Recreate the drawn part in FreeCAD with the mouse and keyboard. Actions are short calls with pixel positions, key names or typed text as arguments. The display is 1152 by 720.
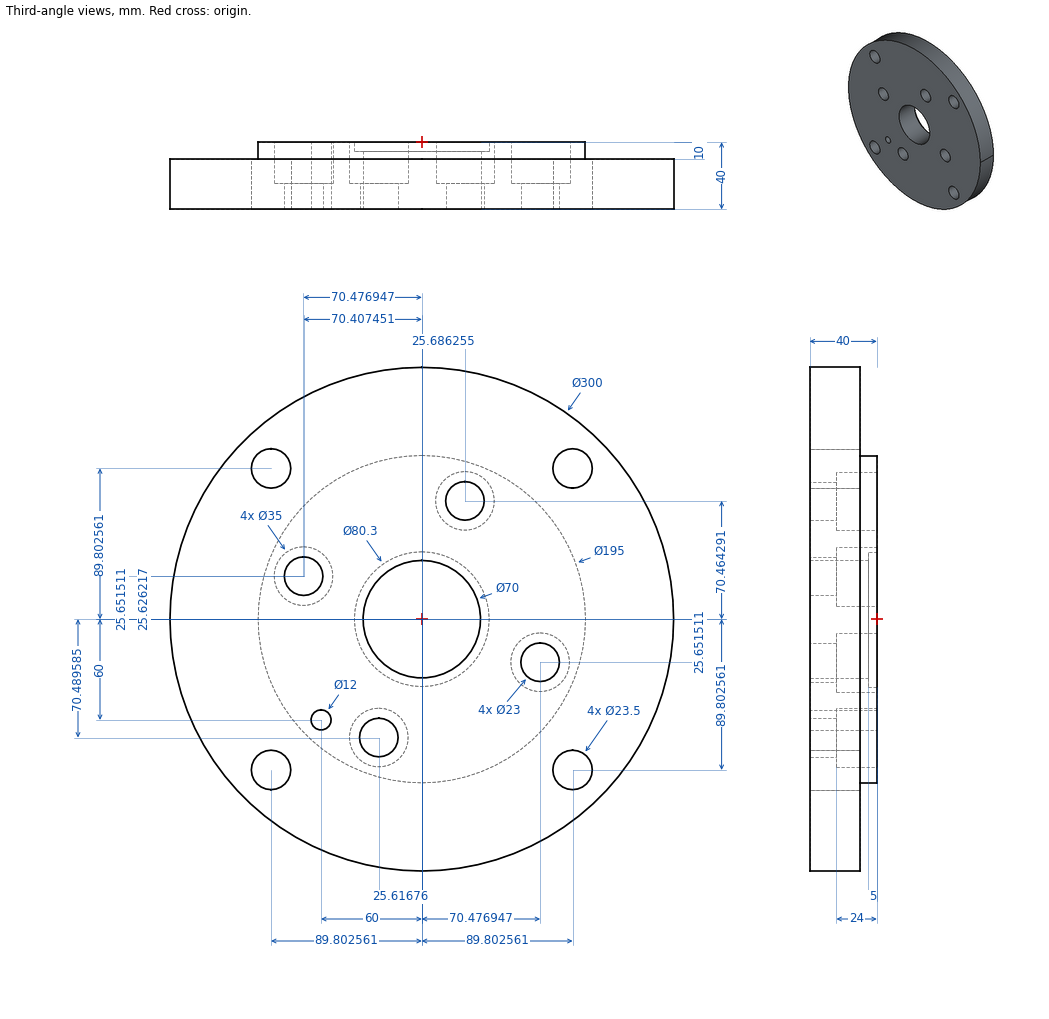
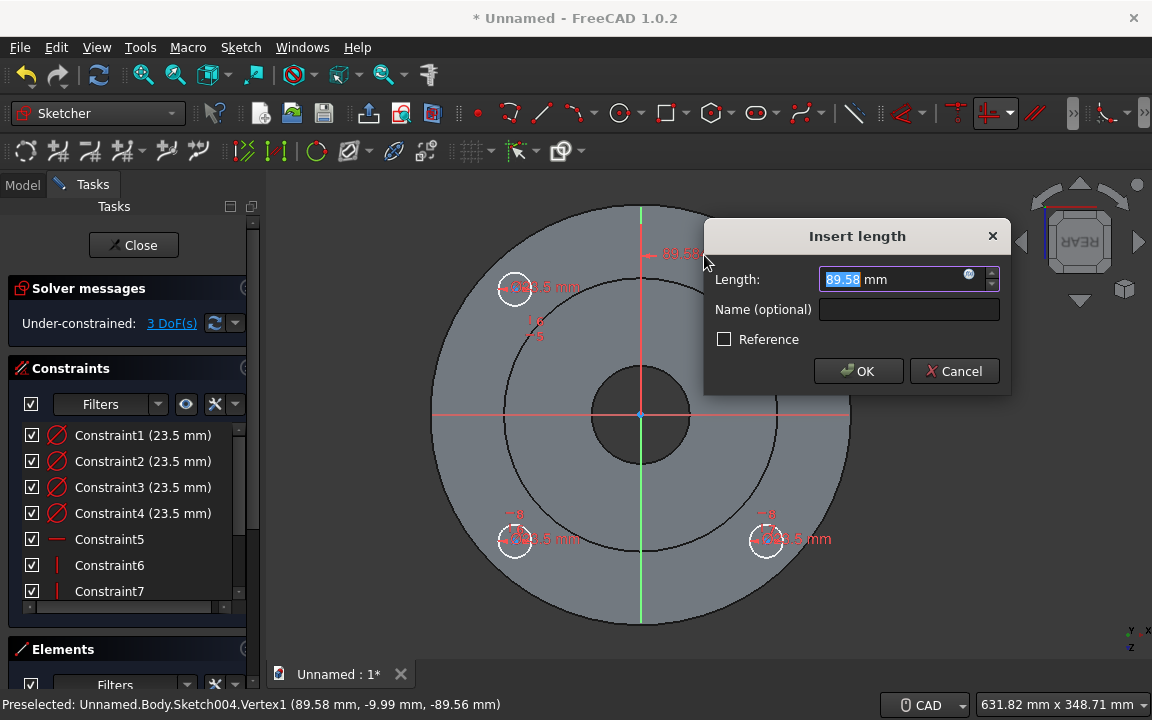
text(89.802561)
key(Return)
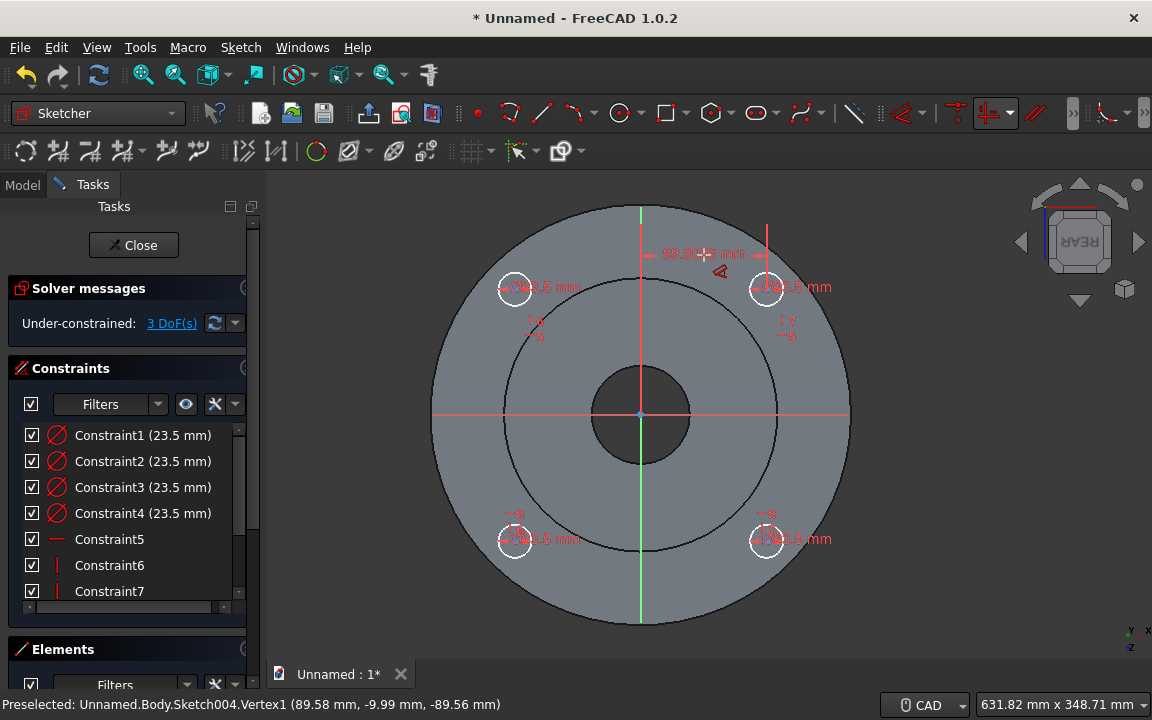
click(767, 289)
click(801, 352)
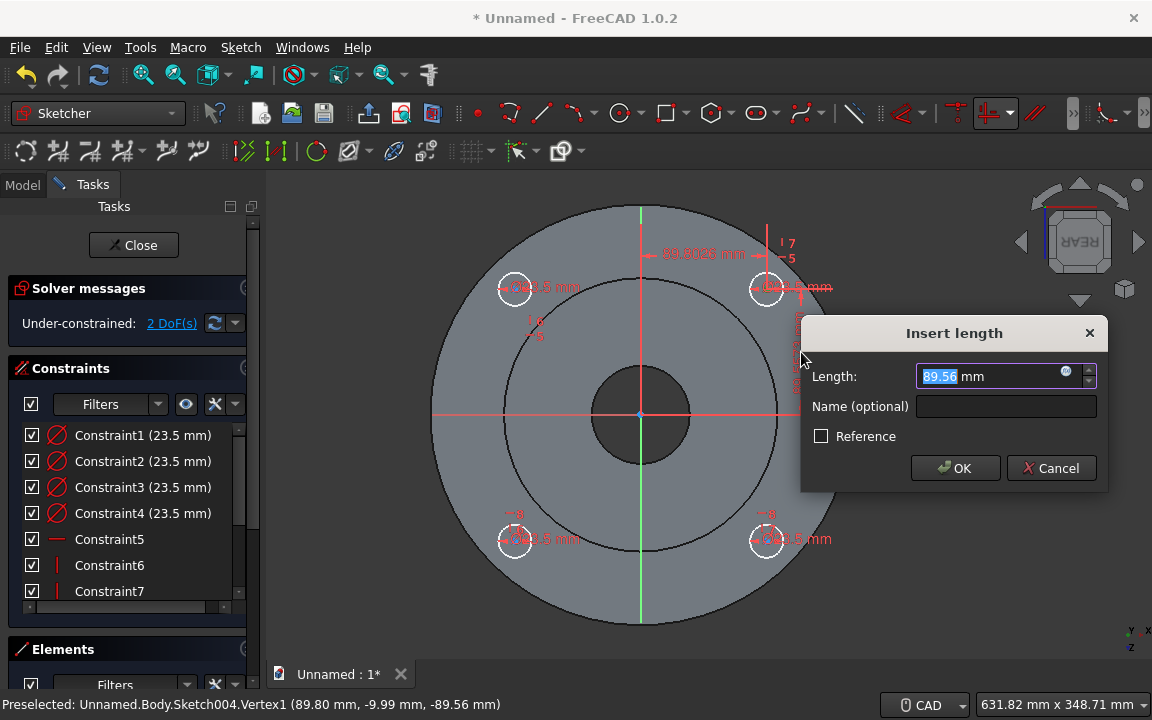
text(89.802561)
key(Return)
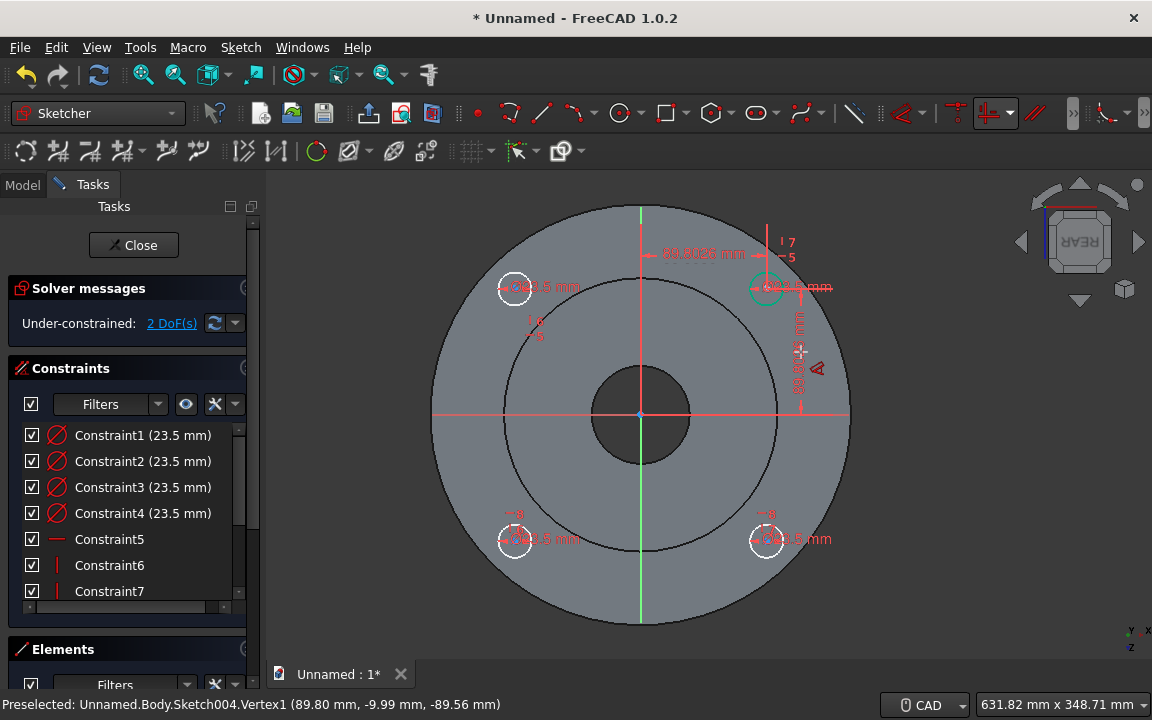
click(515, 289)
click(578, 255)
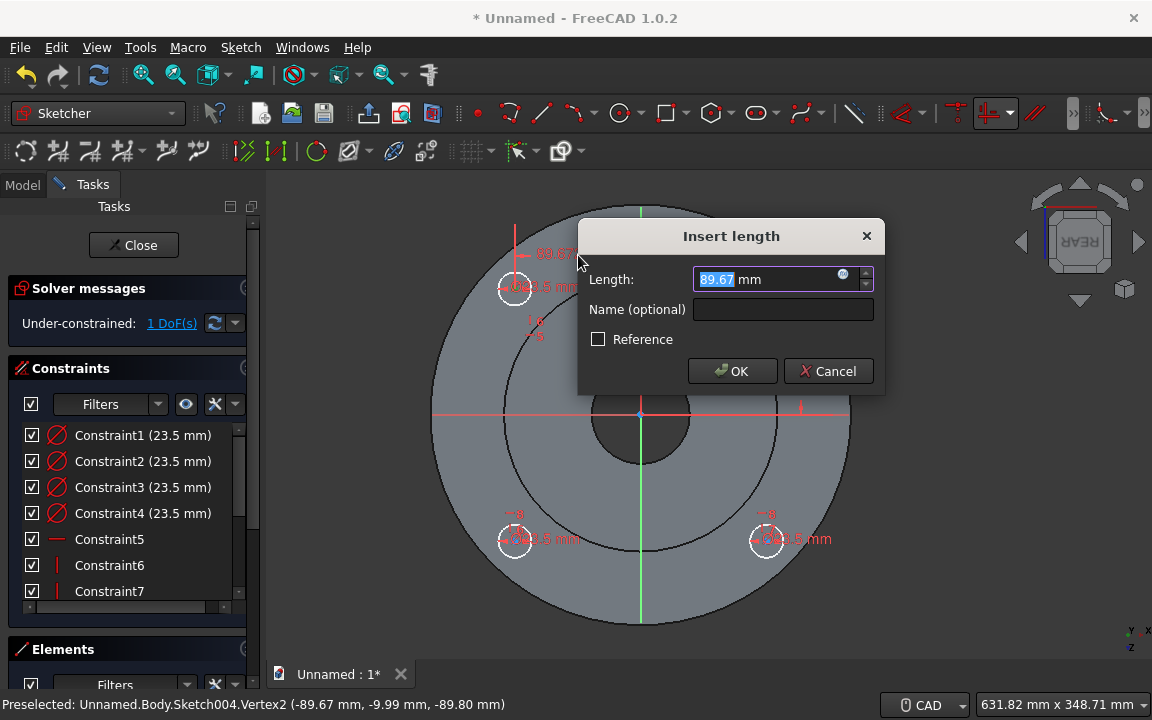
text(89.802561)
key(Return)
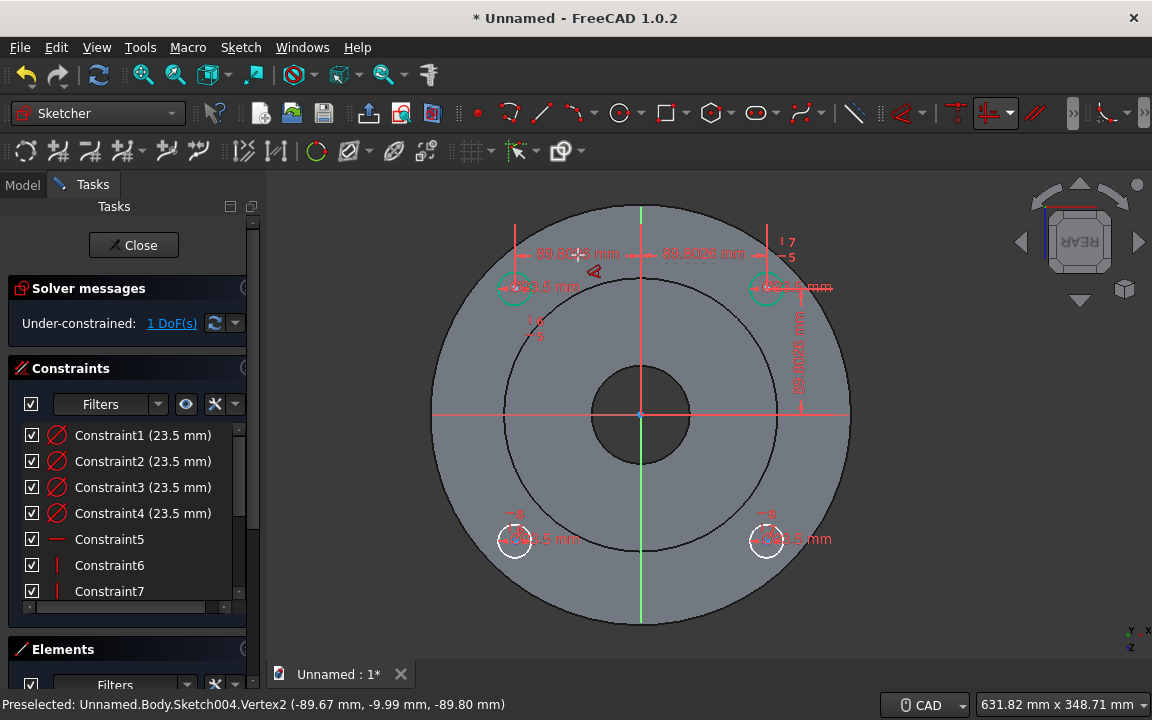
click(515, 541)
click(481, 478)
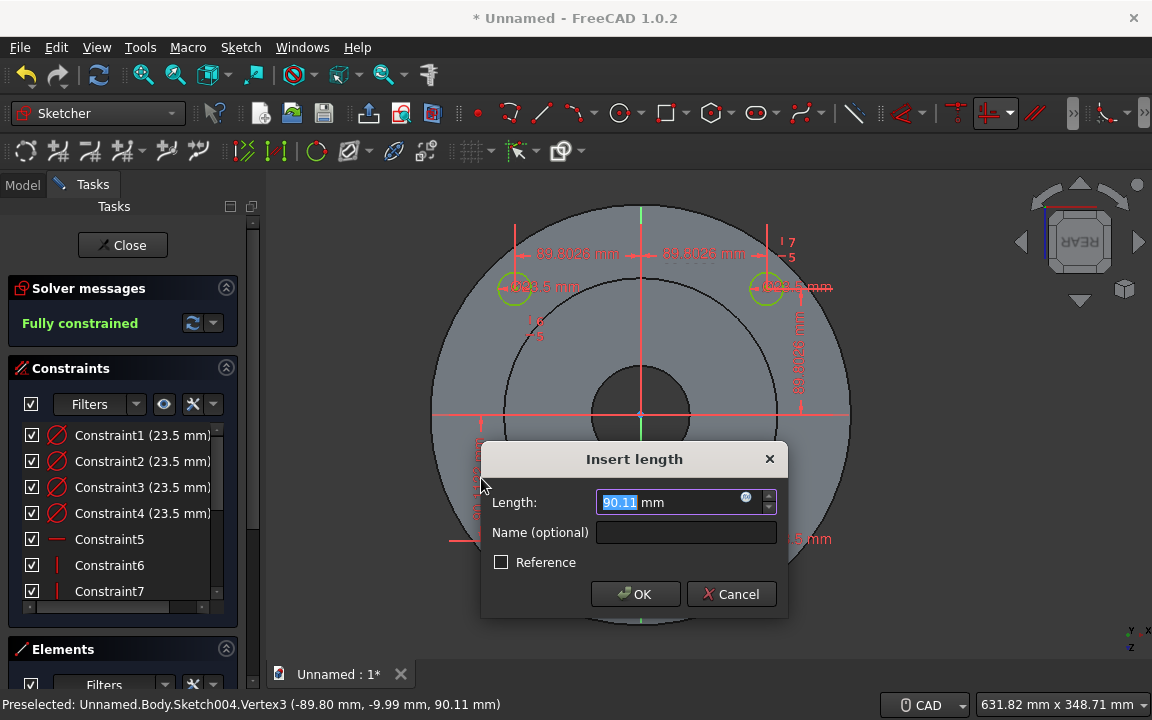
text(89.802561)
key(Return)
key(Escape)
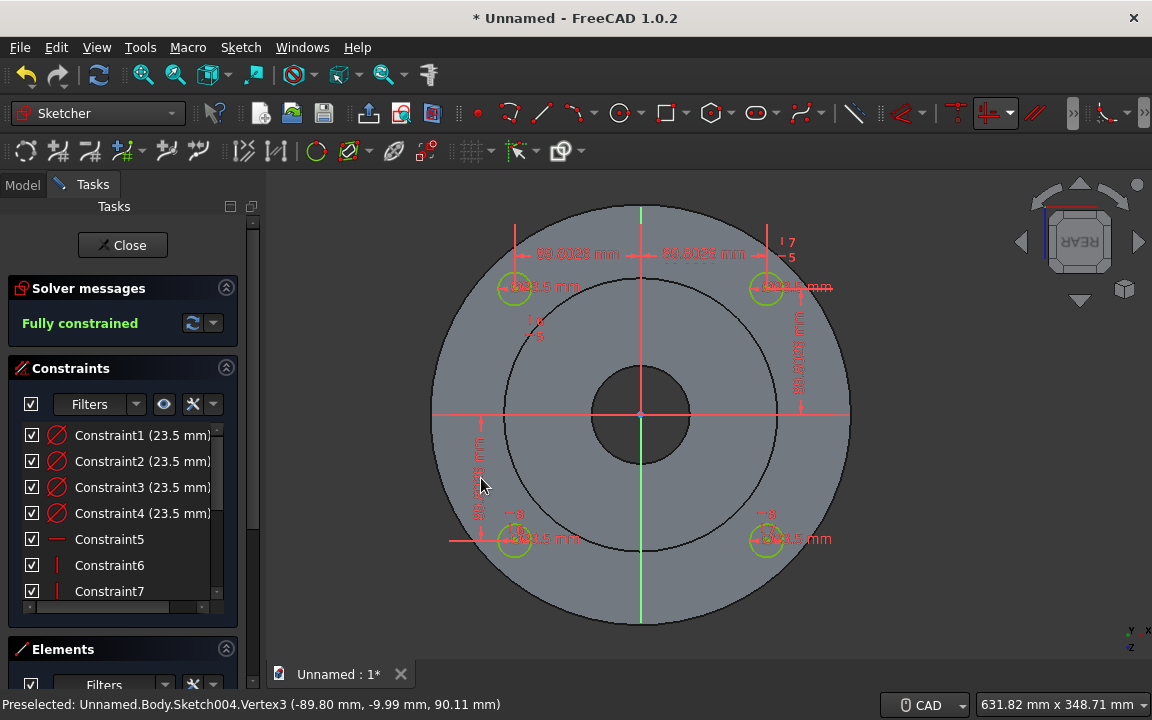
click(123, 245)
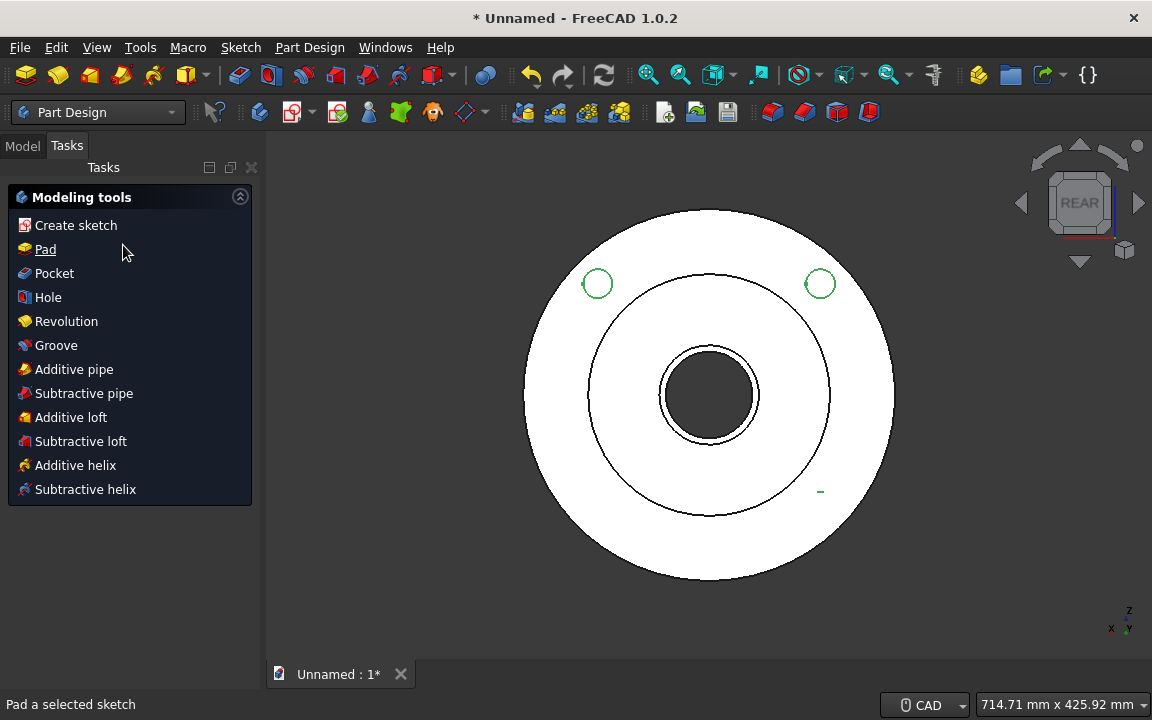
click(240, 76)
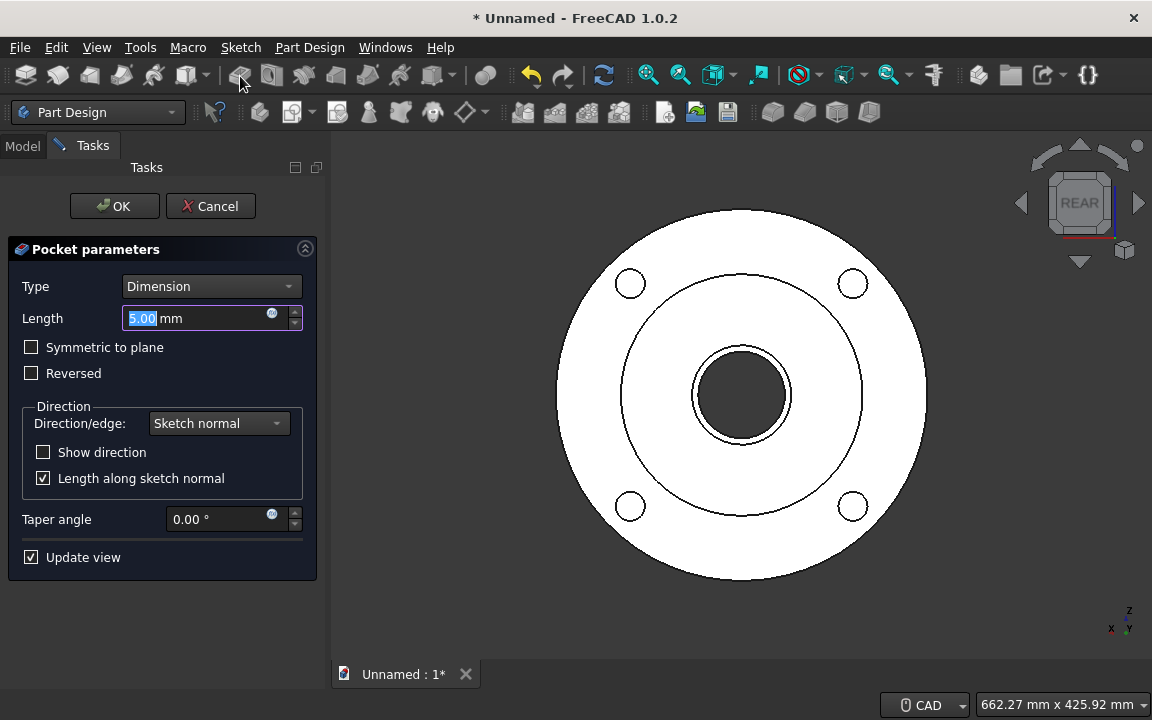
click(212, 286)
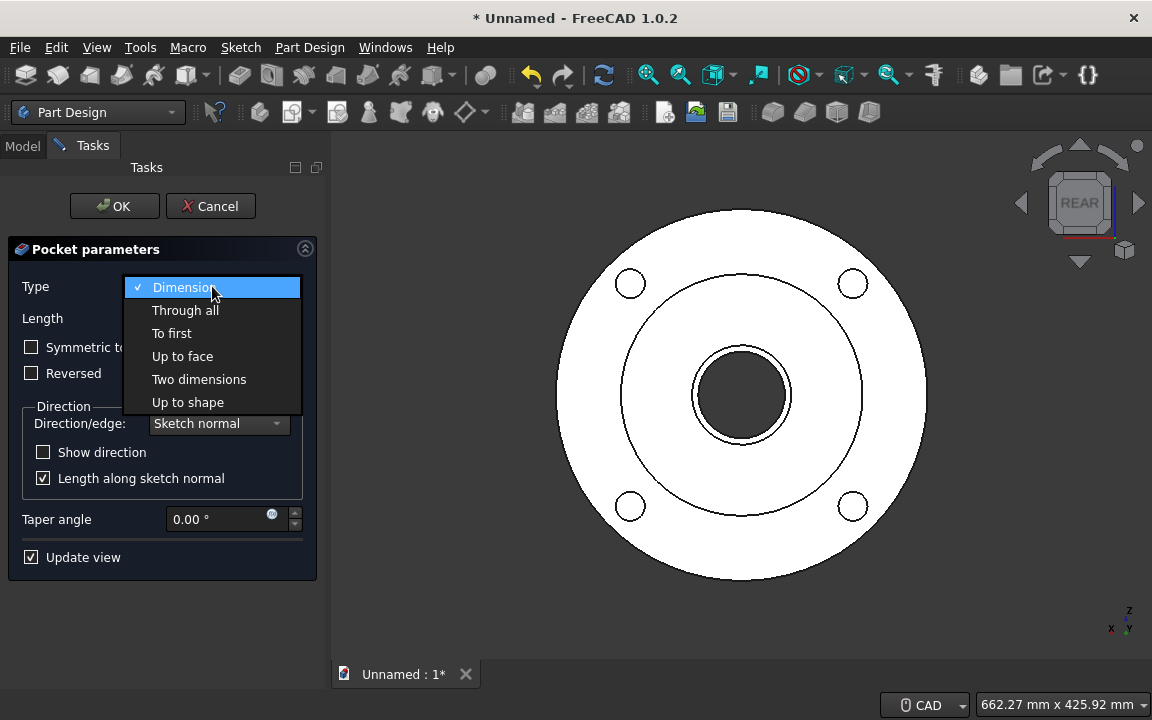
click(212, 310)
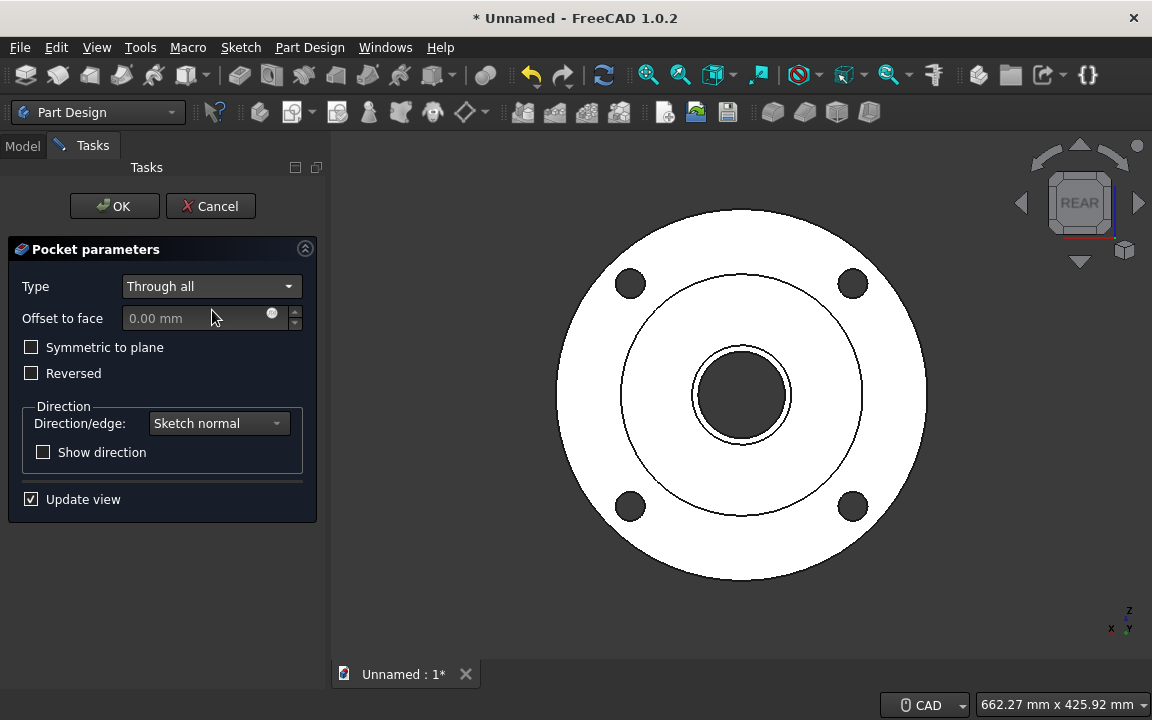
click(115, 206)